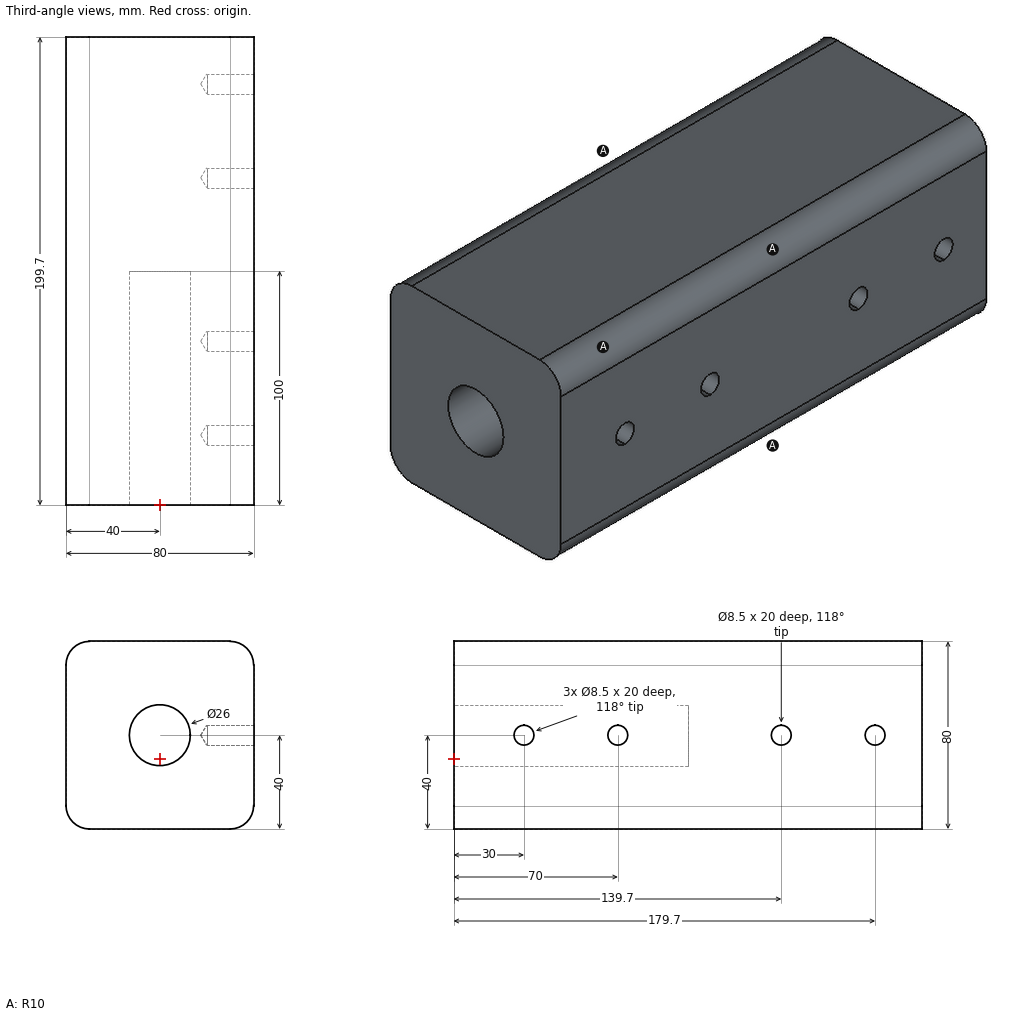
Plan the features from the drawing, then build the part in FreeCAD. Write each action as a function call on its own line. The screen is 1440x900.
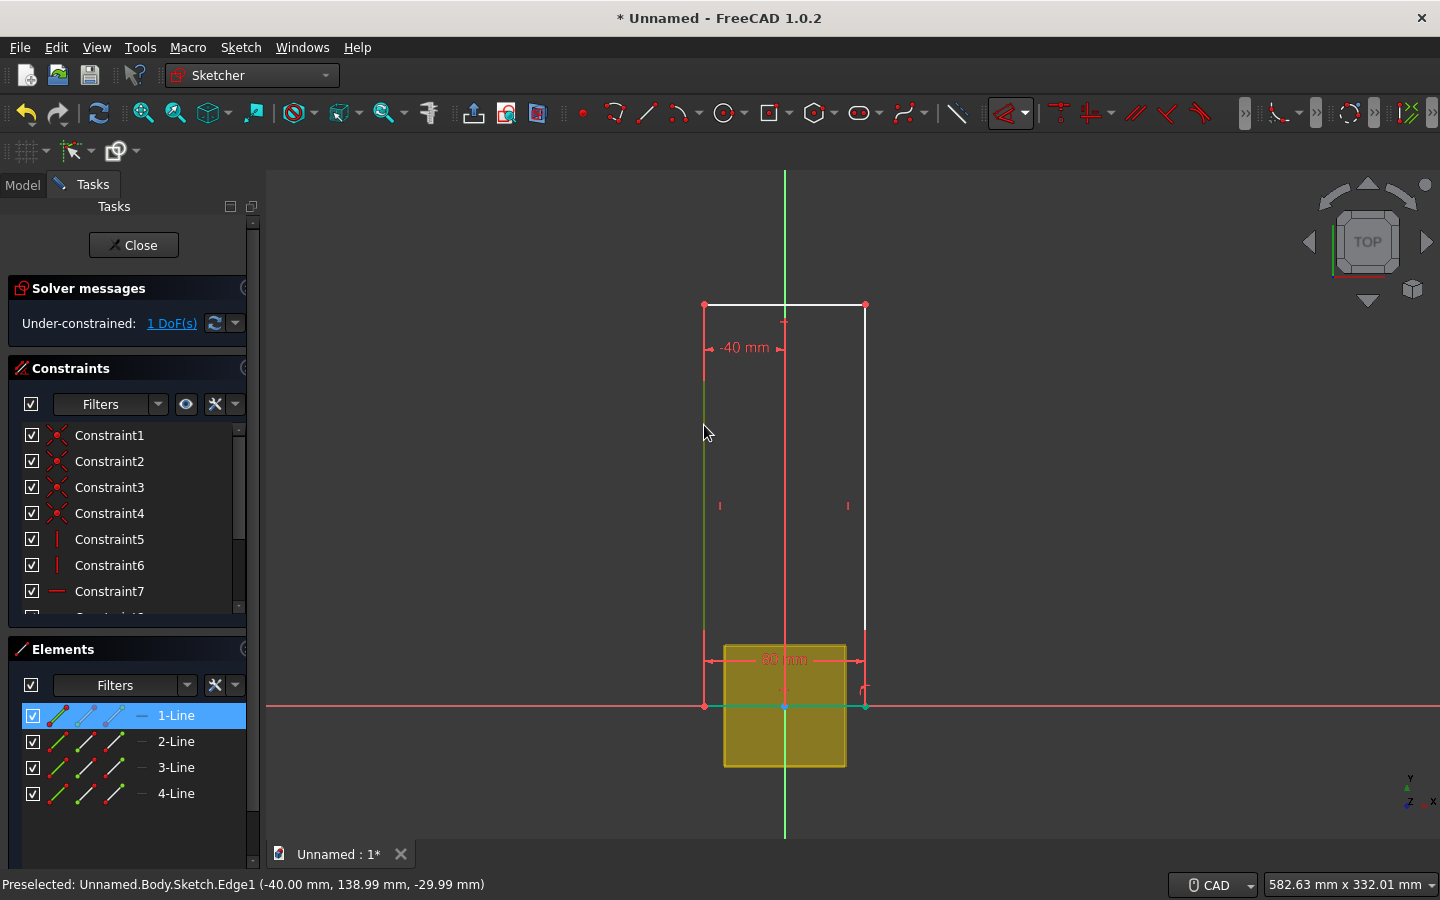
key(i)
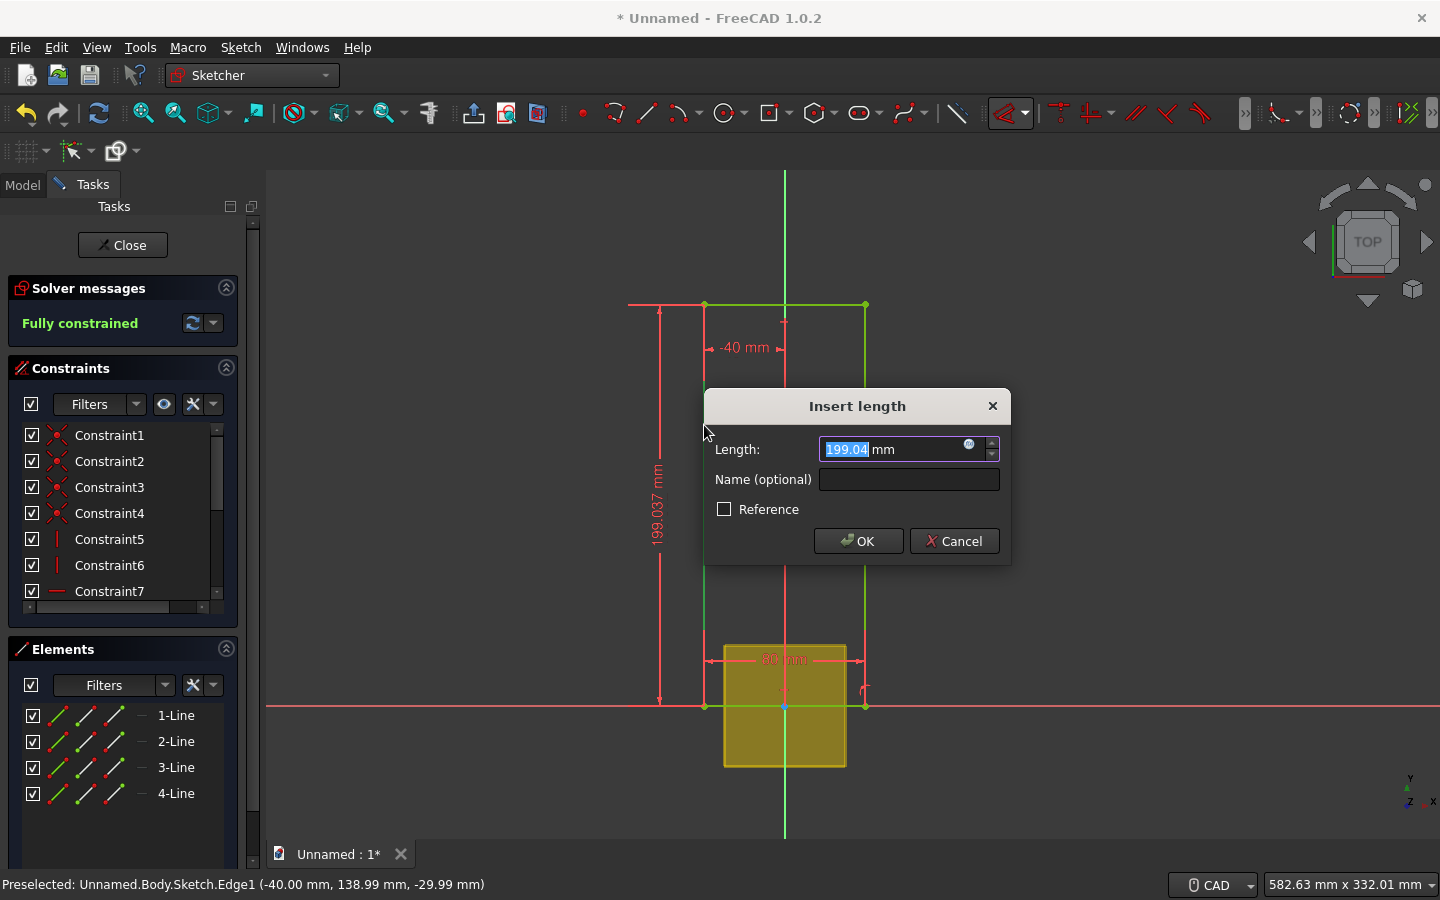
text(199.7)
key(Return)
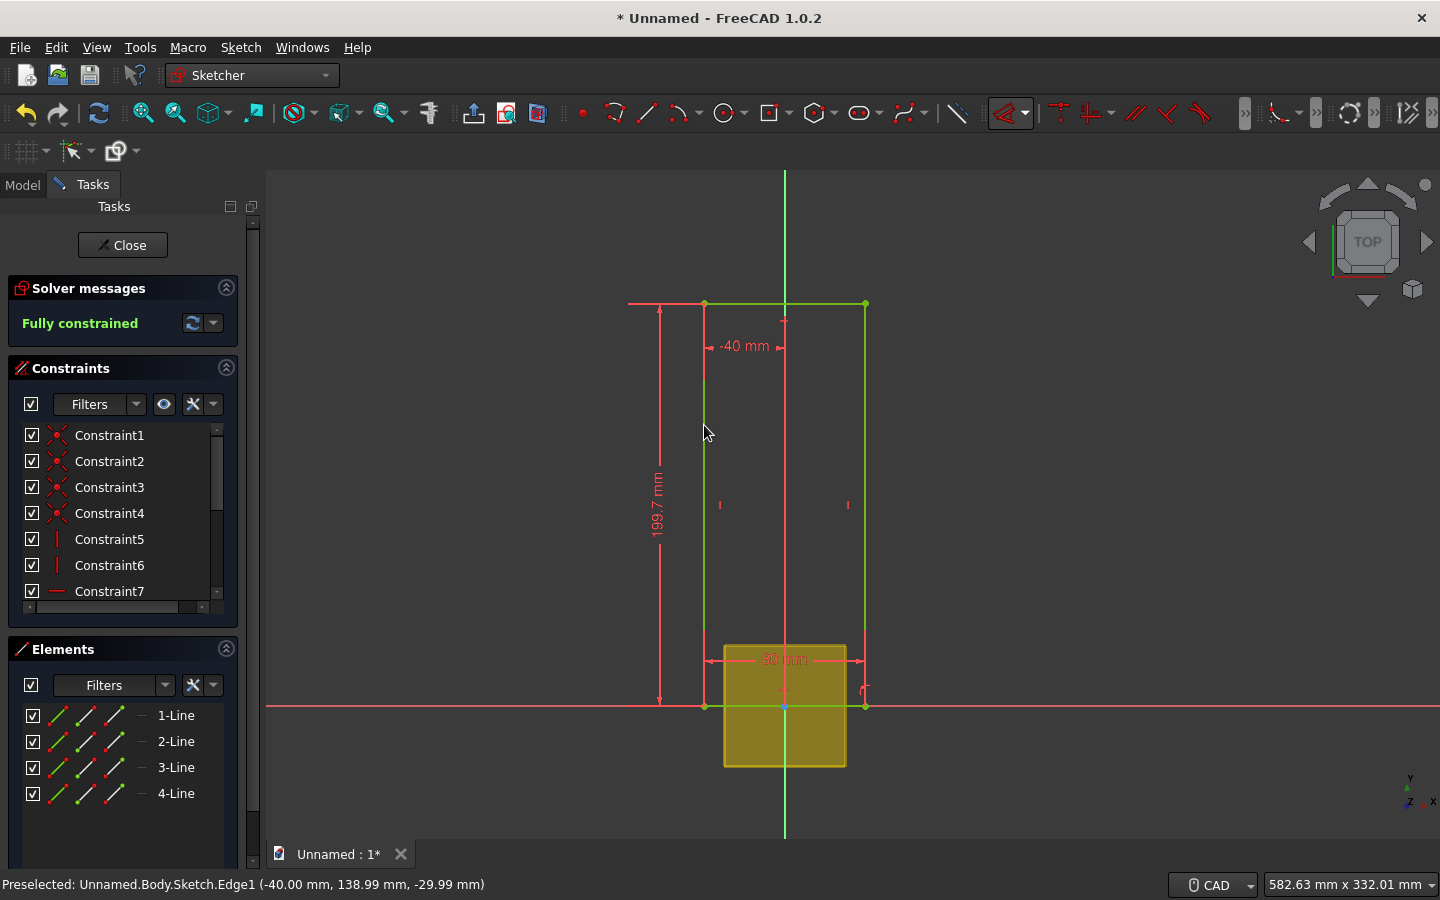
click(123, 245)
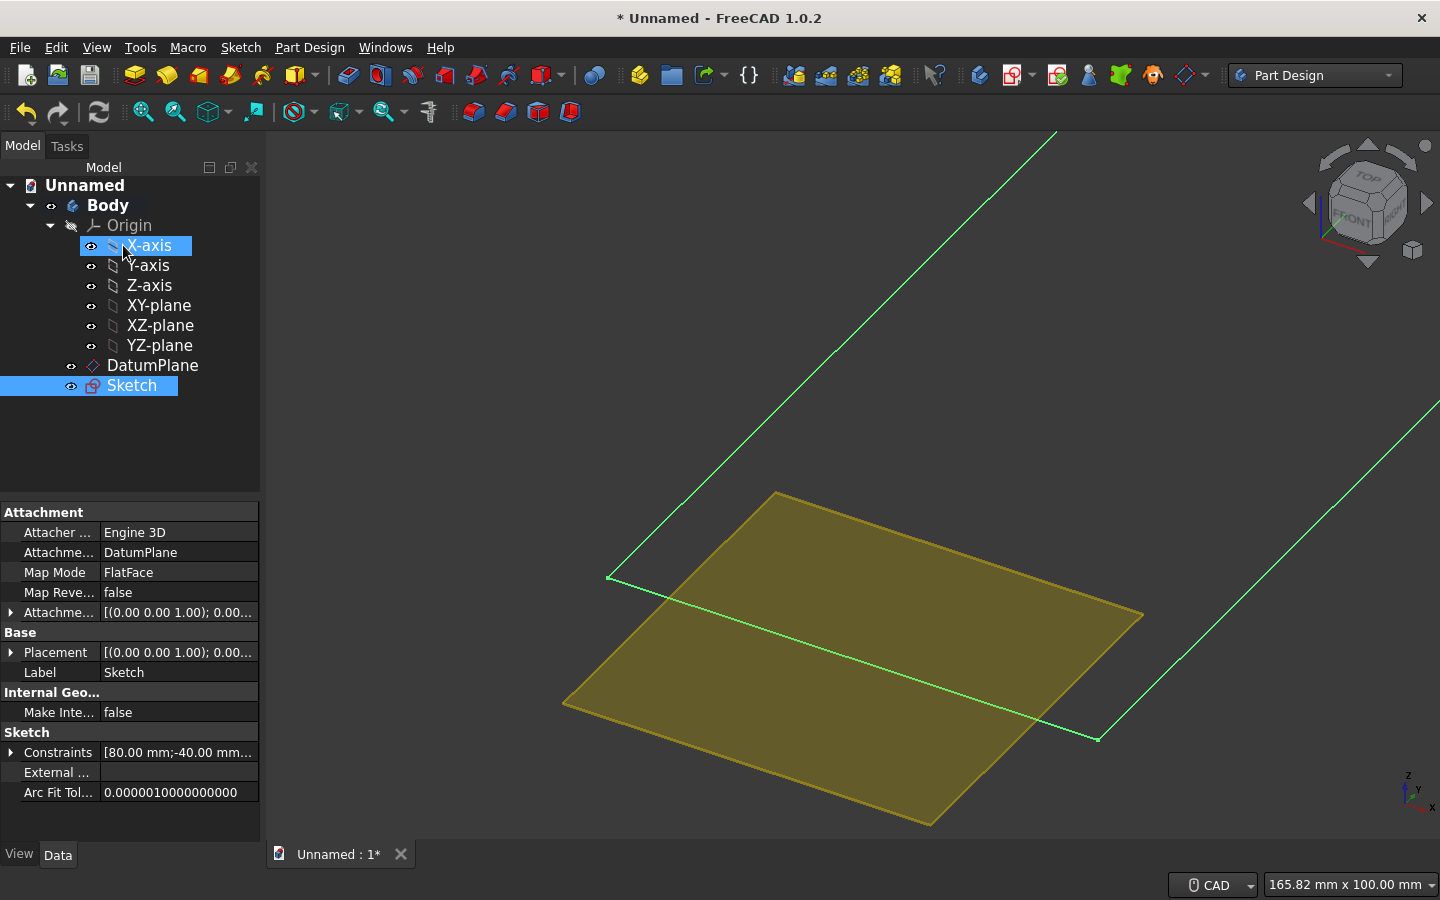
click(136, 76)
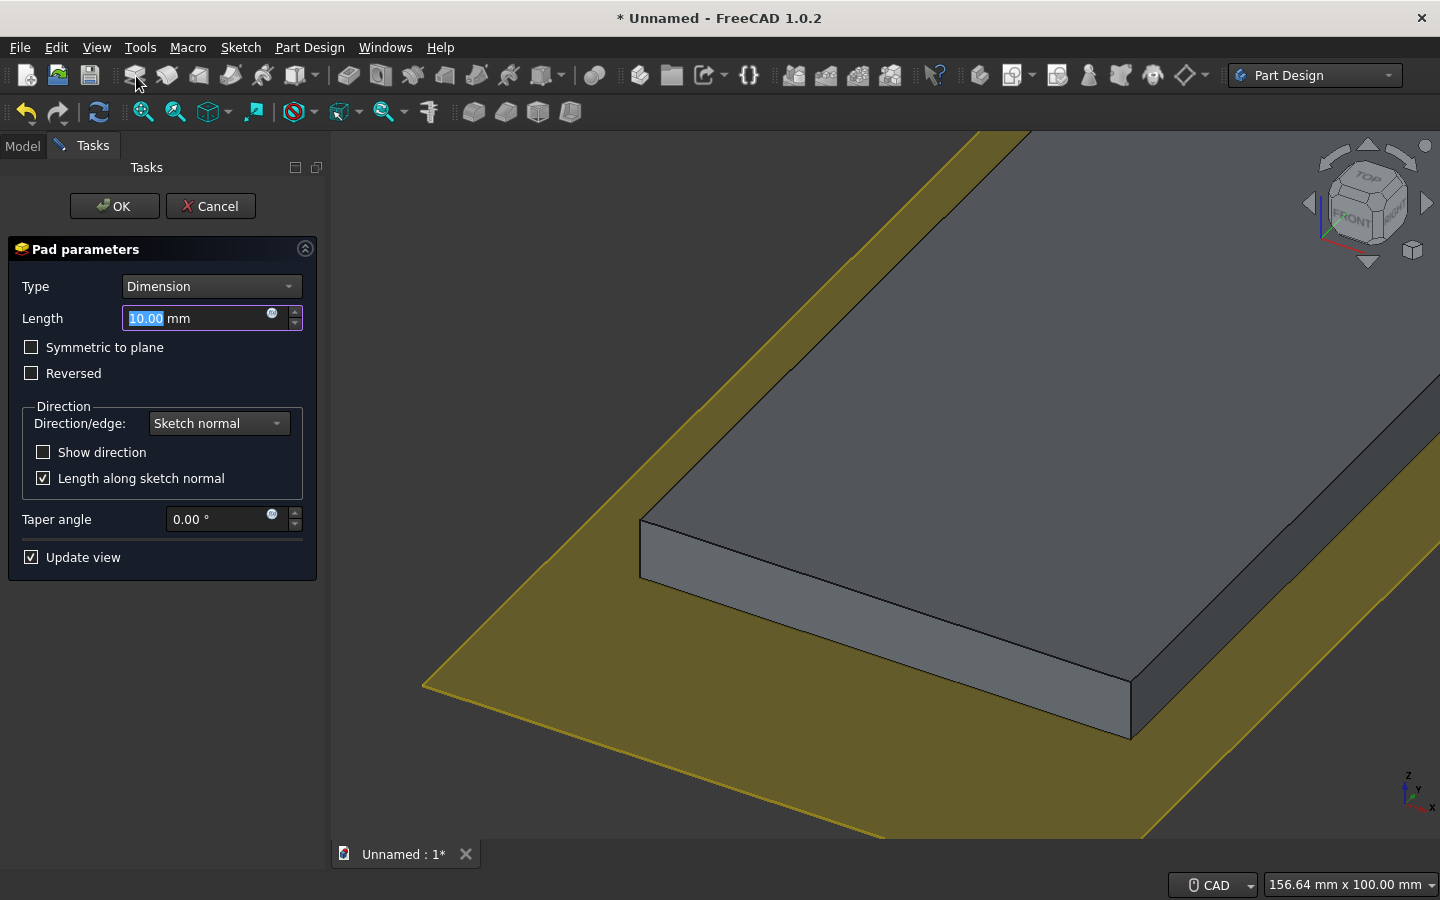
text(80)
key(Tab)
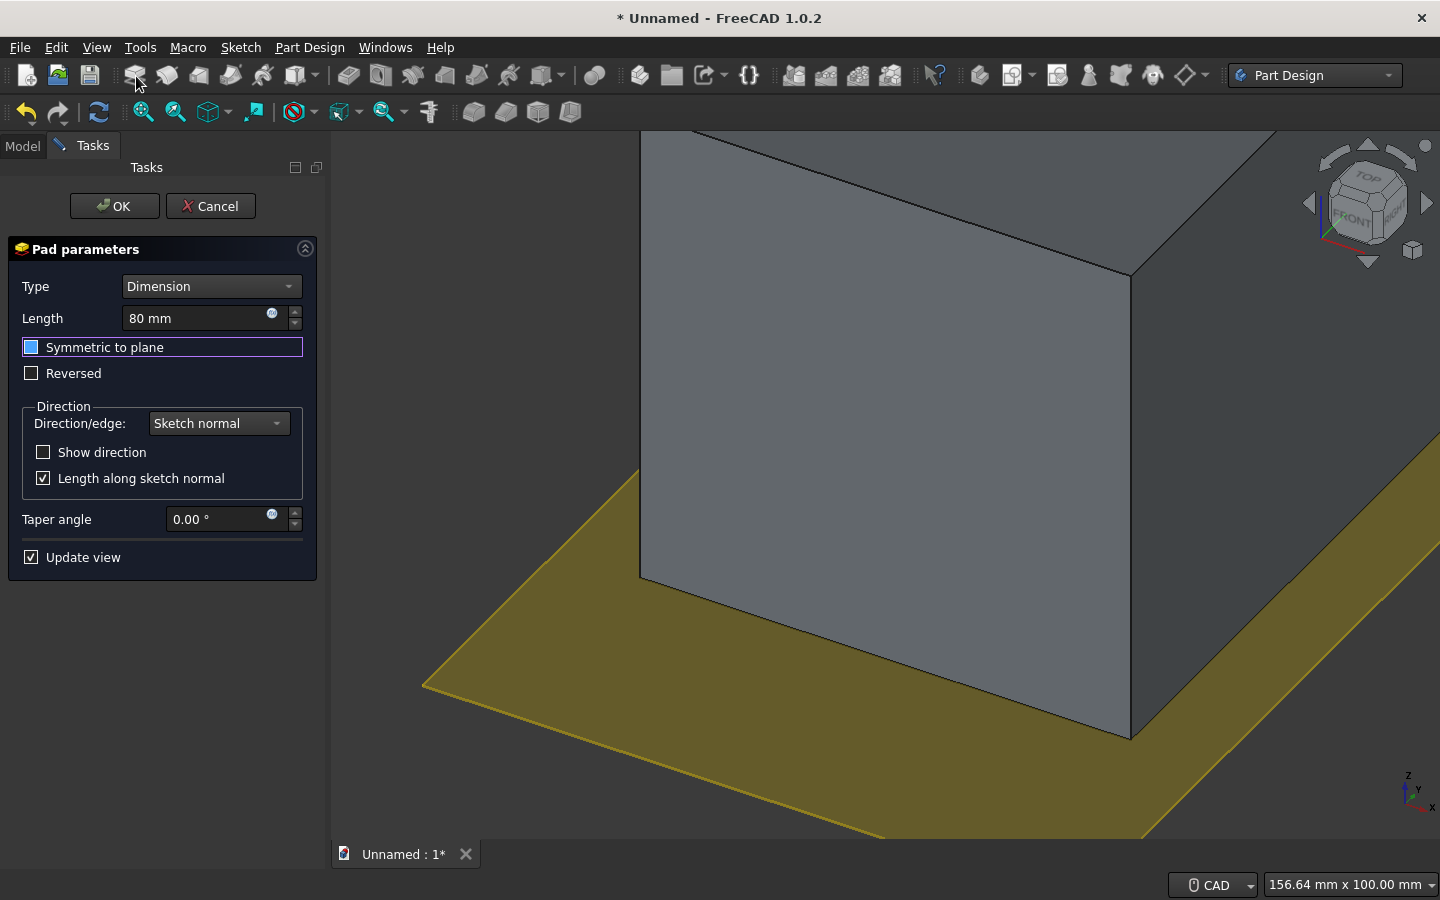
click(115, 206)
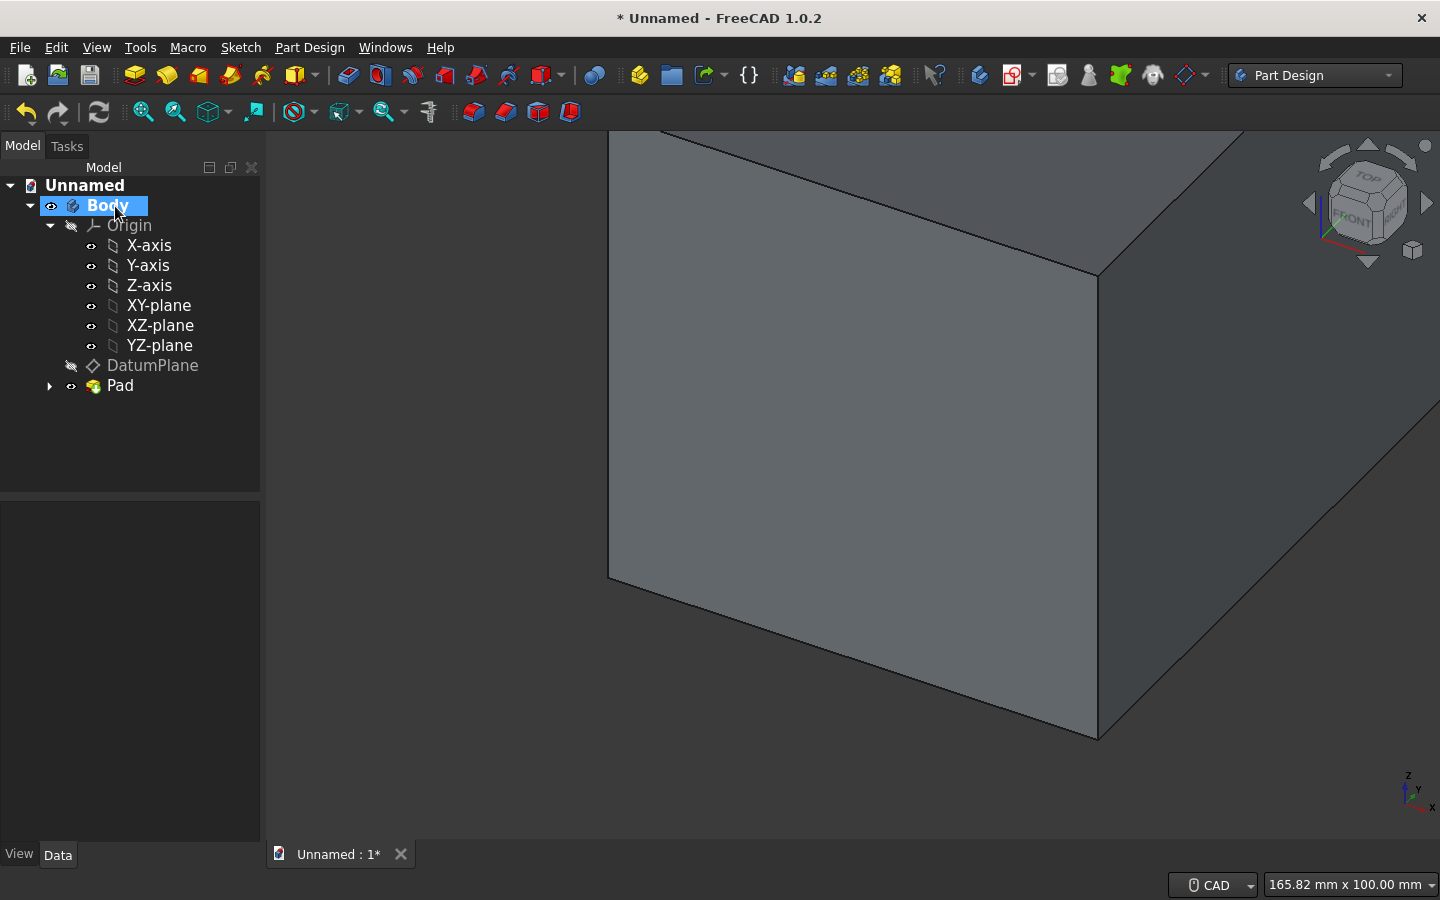
click(144, 112)